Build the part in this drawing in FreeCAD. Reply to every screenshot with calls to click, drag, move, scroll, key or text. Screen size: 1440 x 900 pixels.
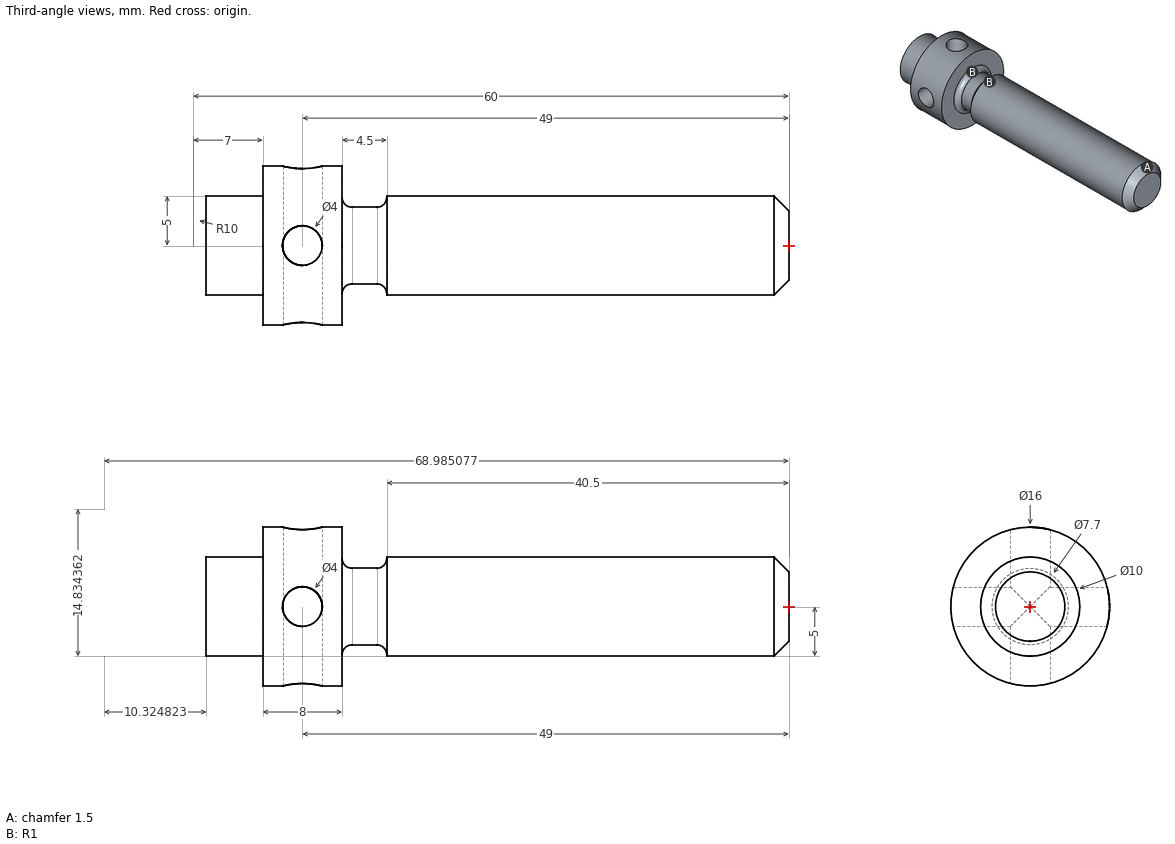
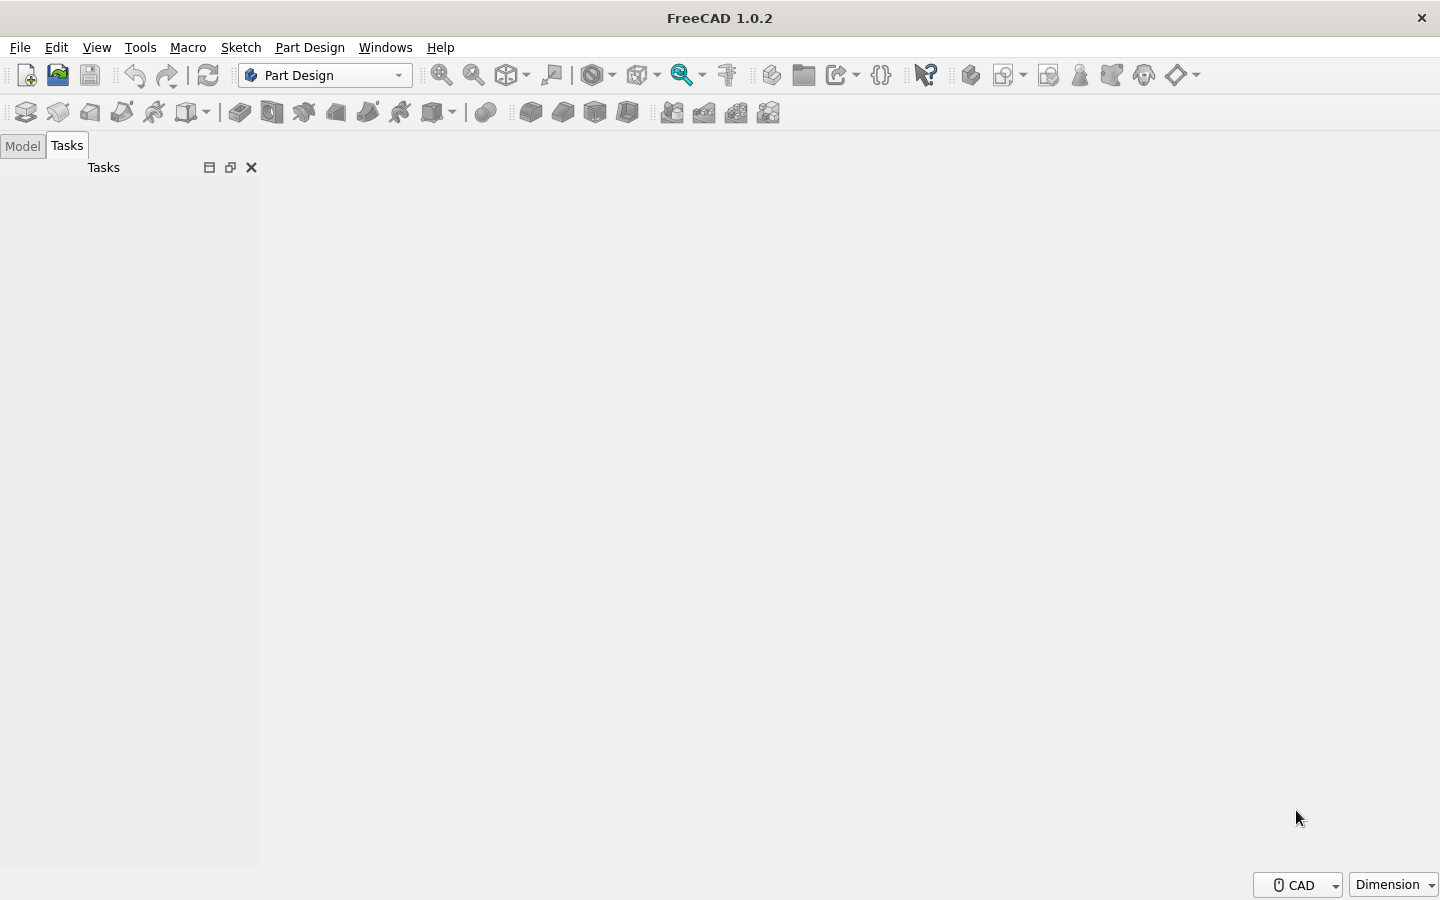
click(26, 76)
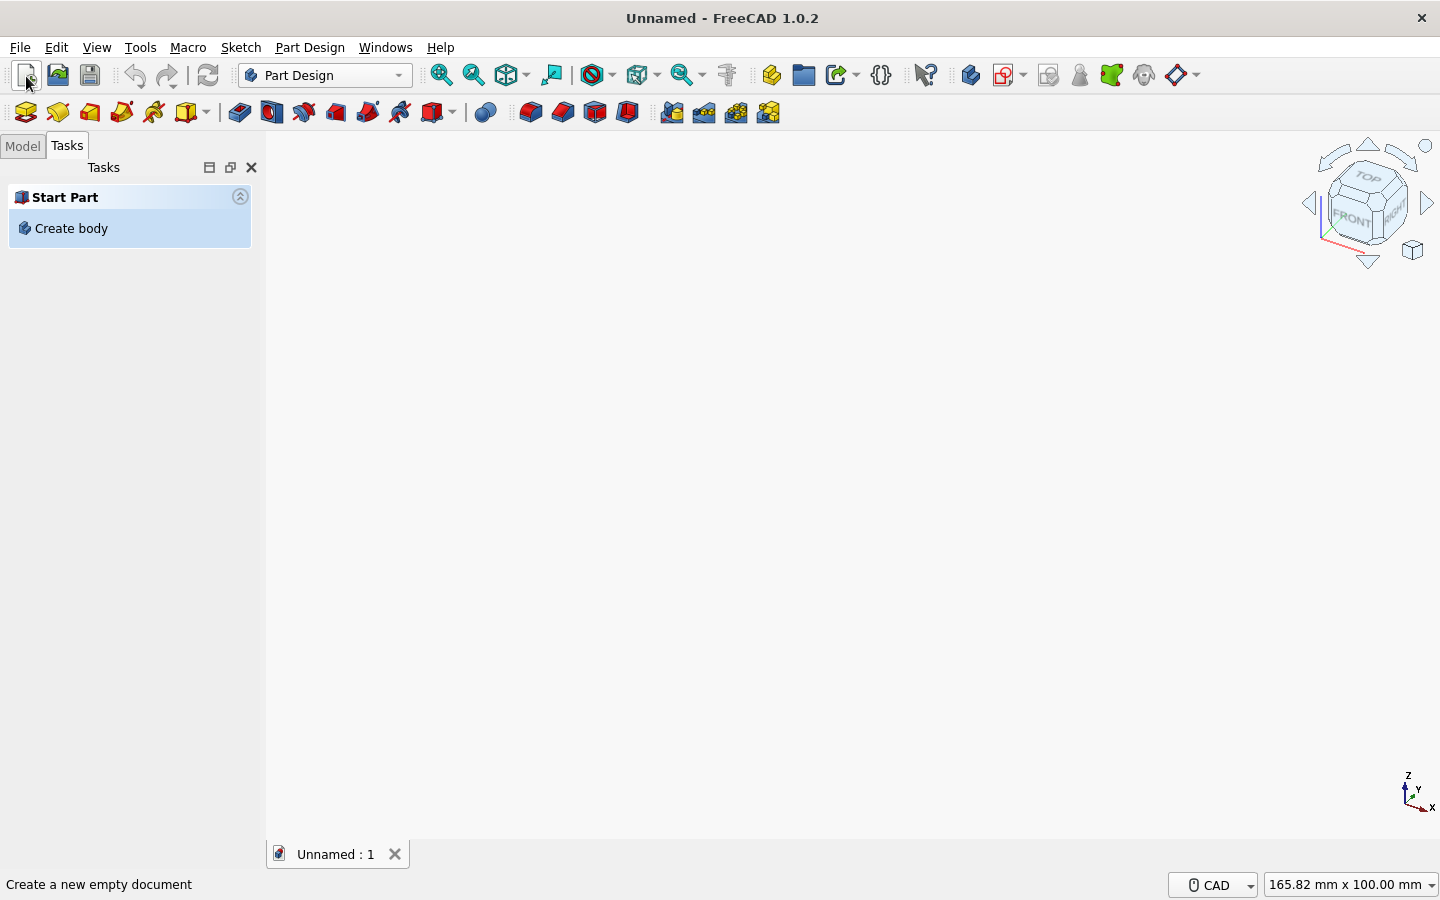
click(1004, 76)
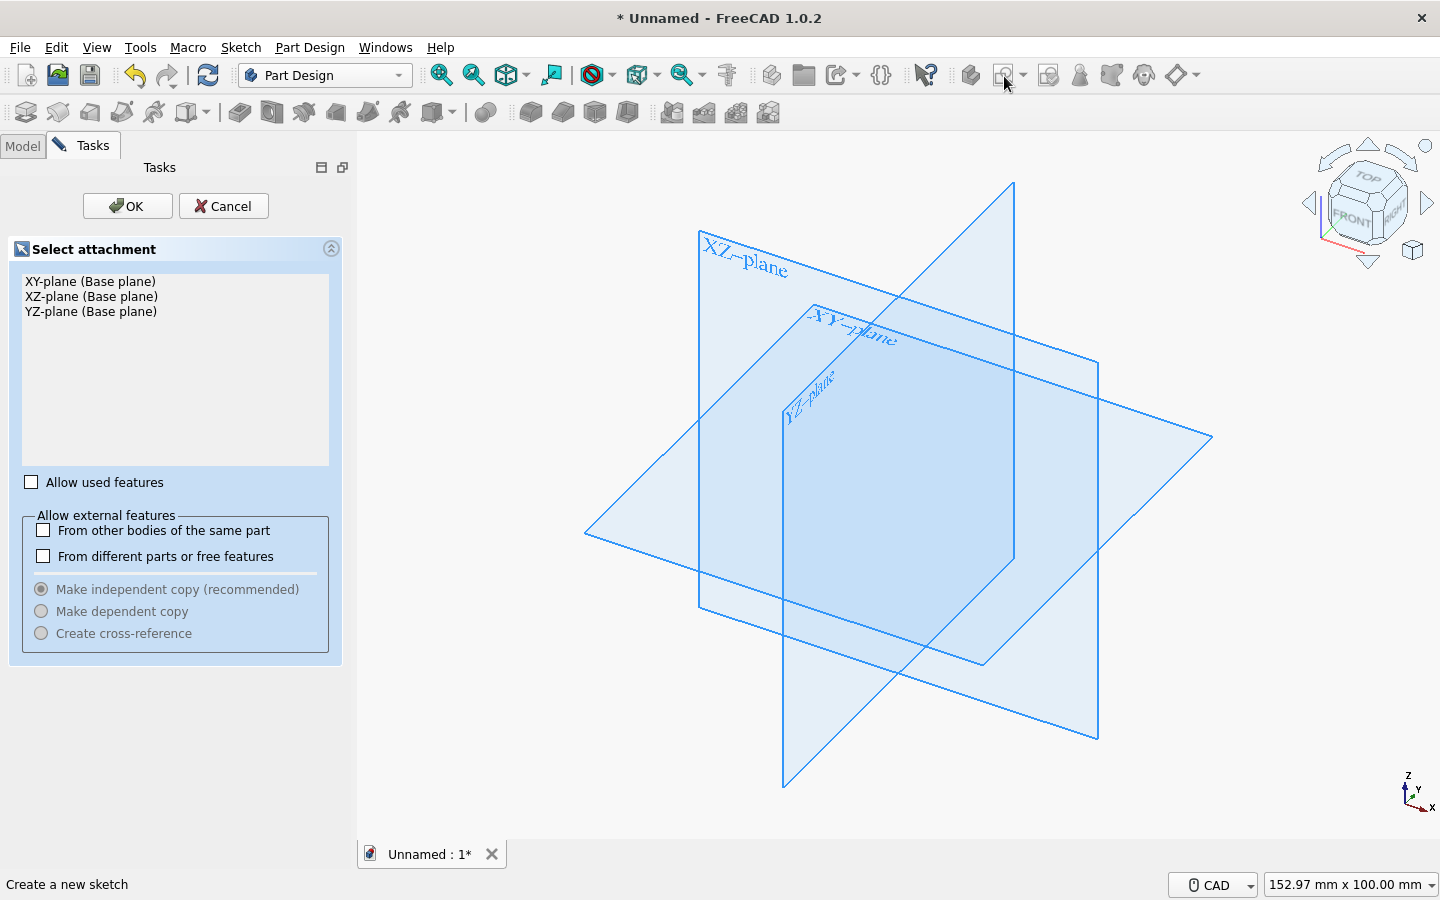
click(82, 312)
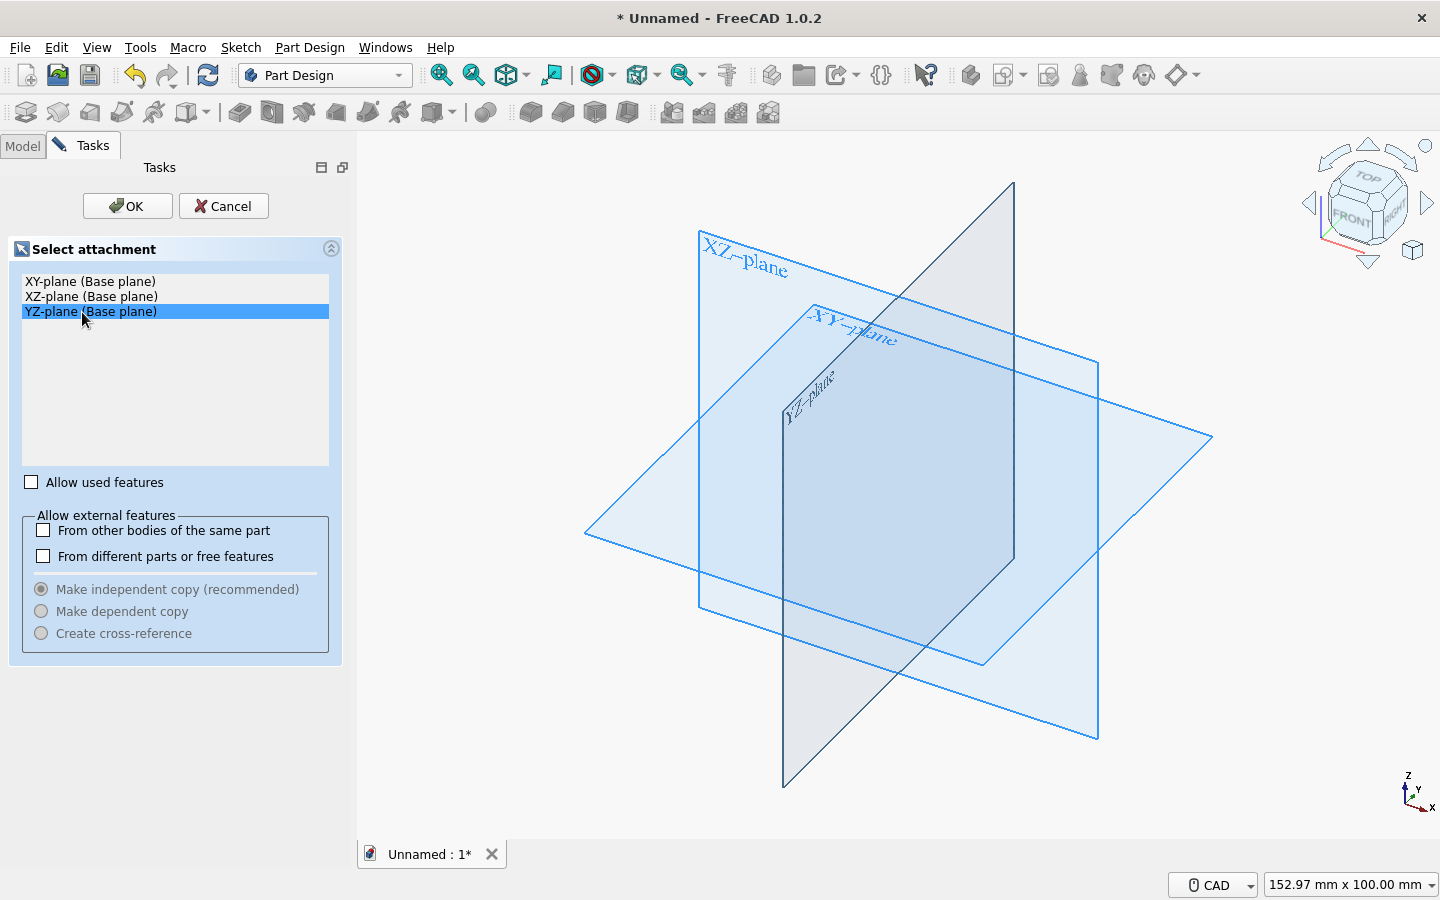
click(128, 206)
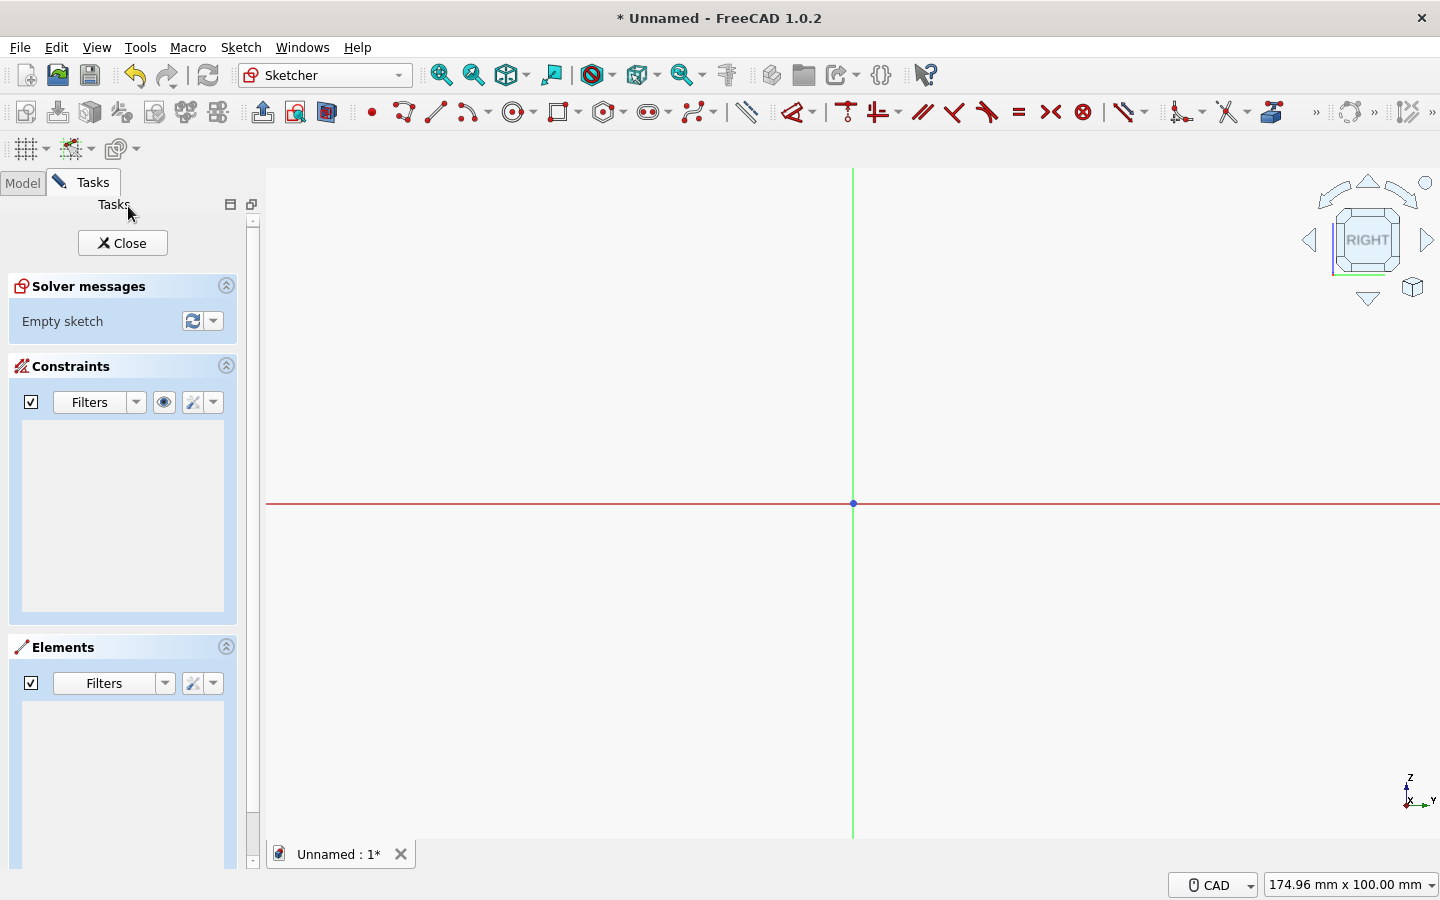
scroll(867, 504, up, 9)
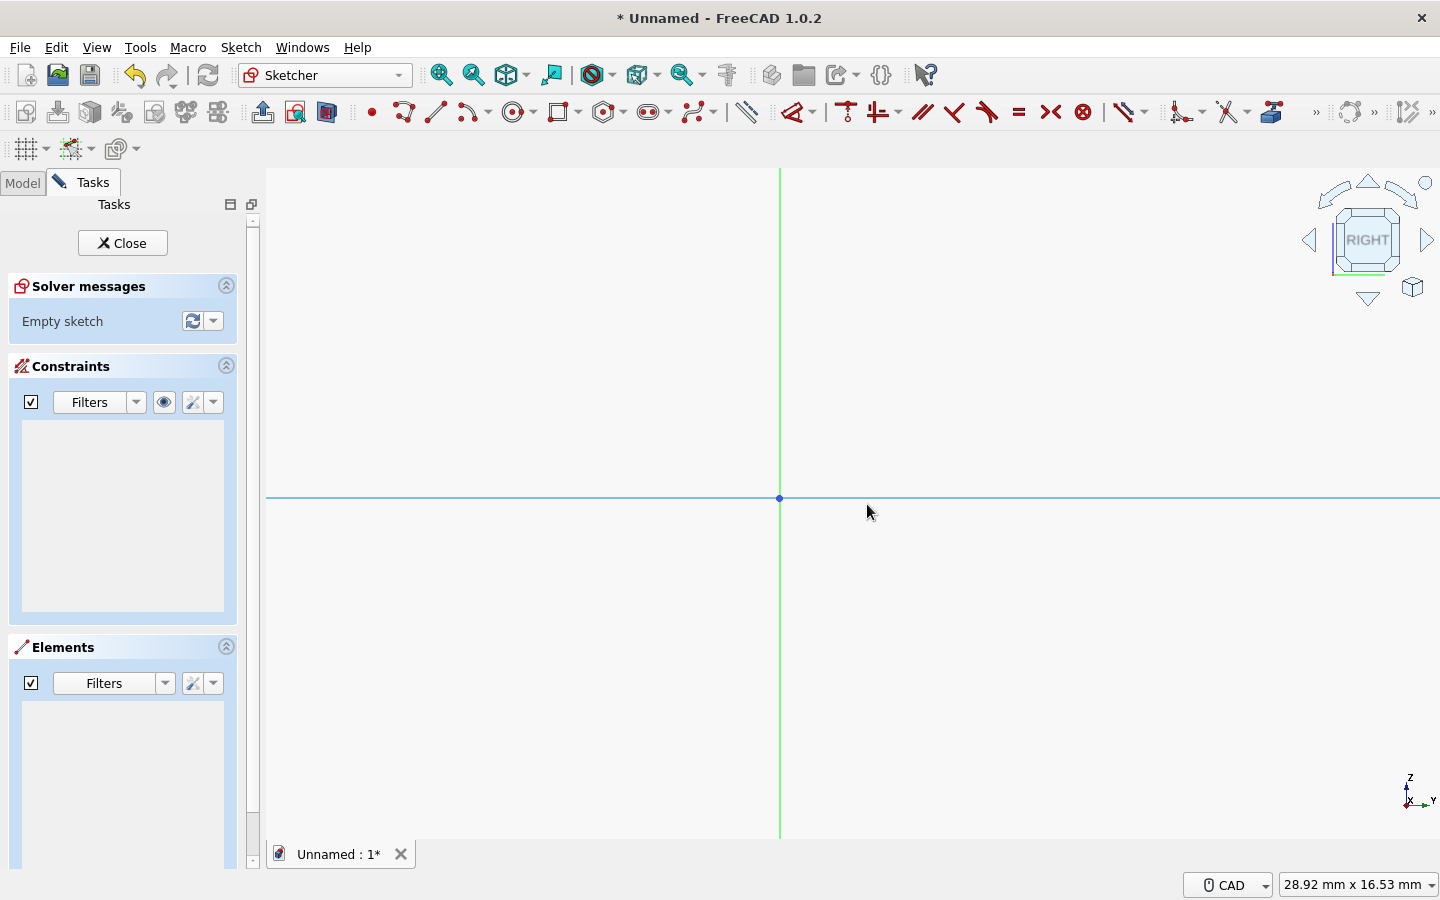
key(g)
key(c)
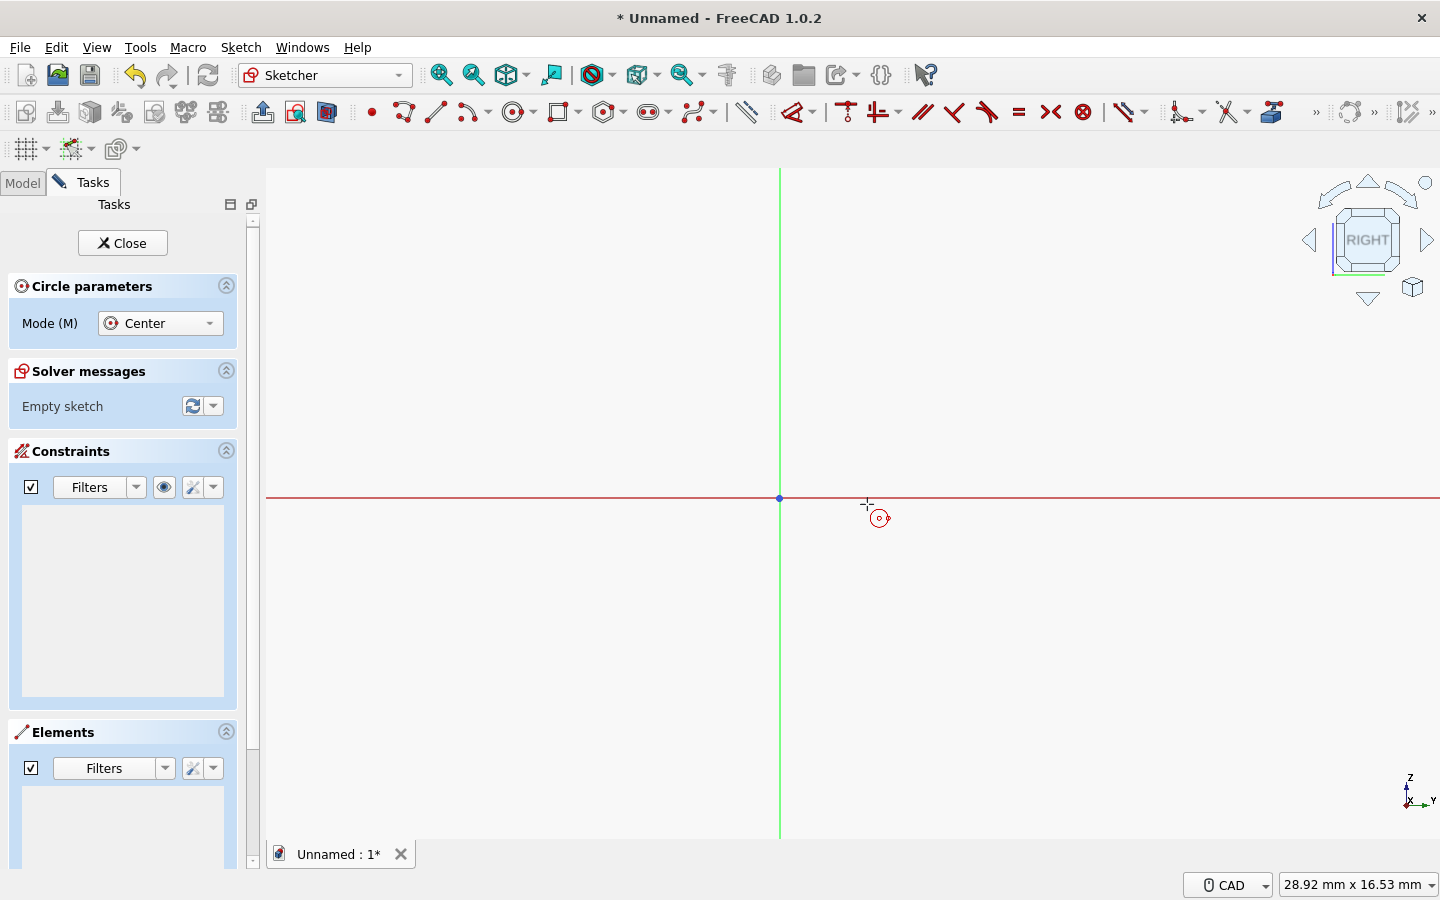
click(780, 498)
click(923, 355)
key(Escape)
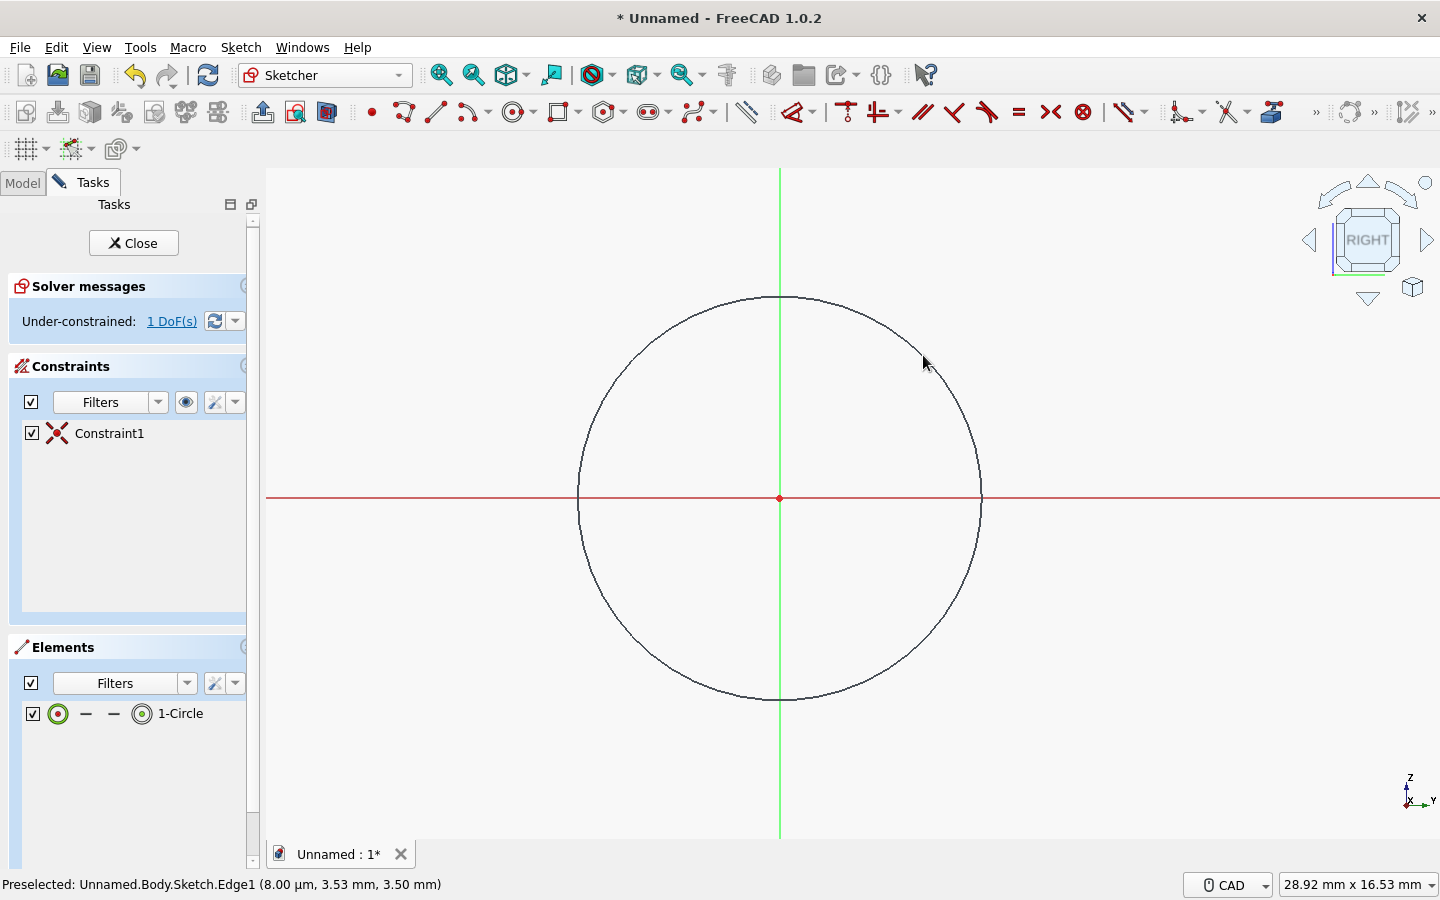
click(792, 112)